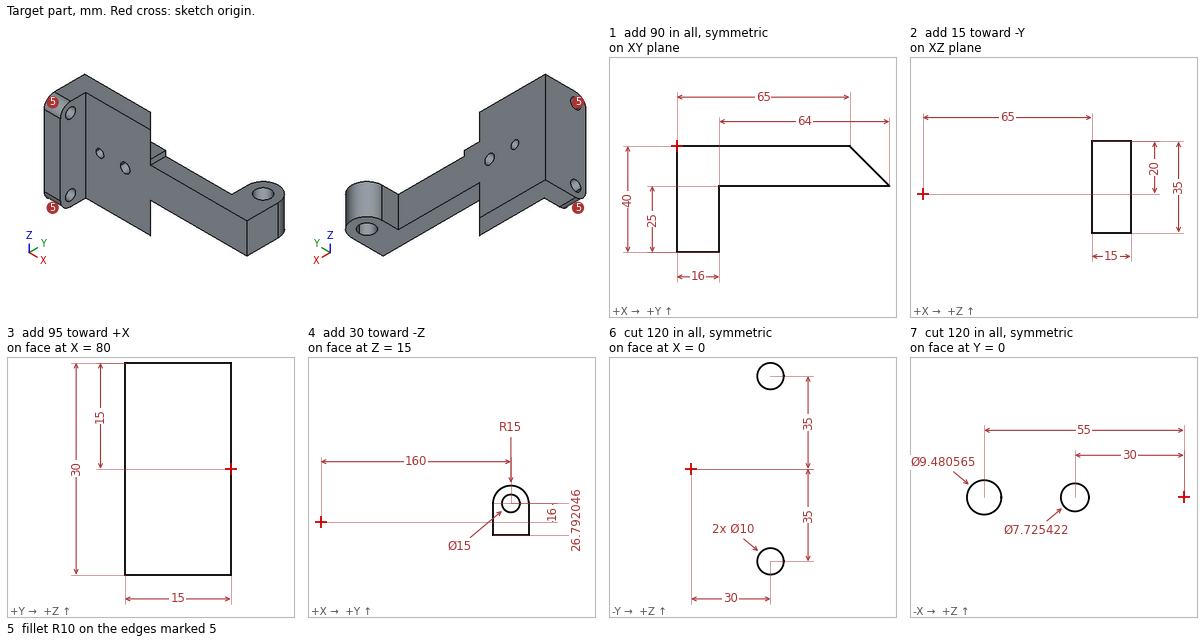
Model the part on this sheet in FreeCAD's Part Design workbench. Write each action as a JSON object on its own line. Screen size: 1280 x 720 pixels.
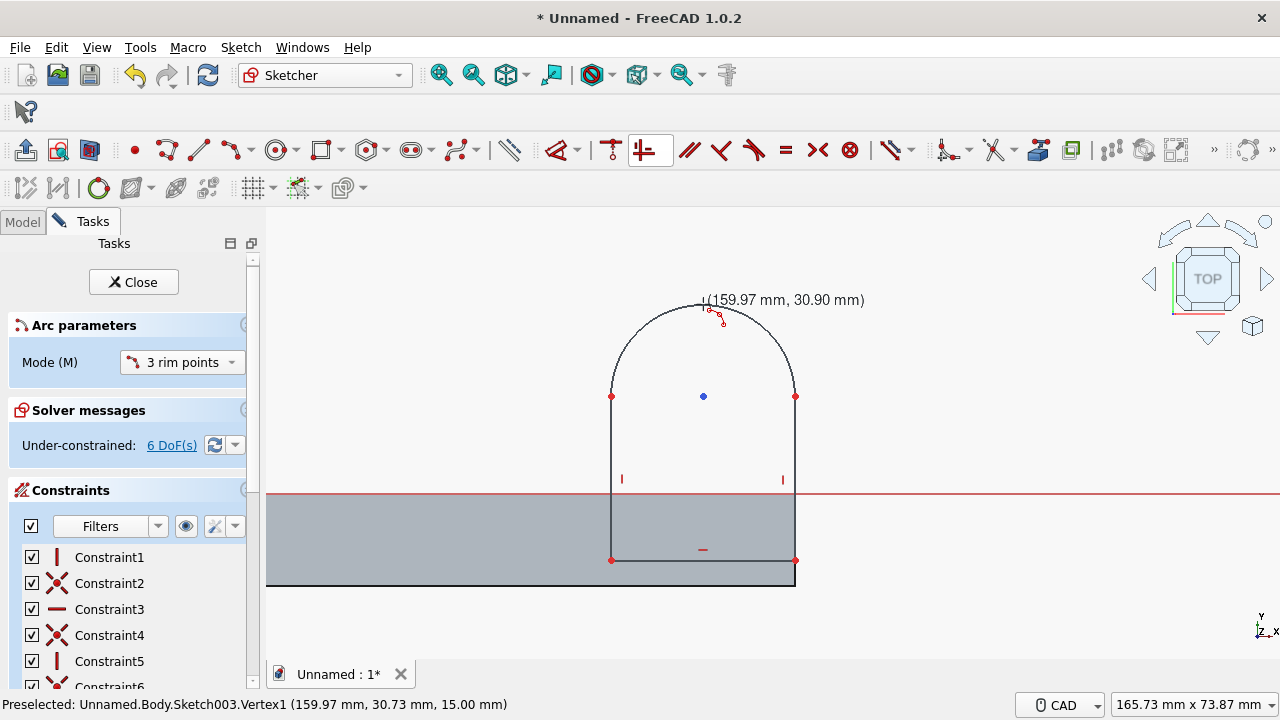
{"action": "key", "text": "g c"}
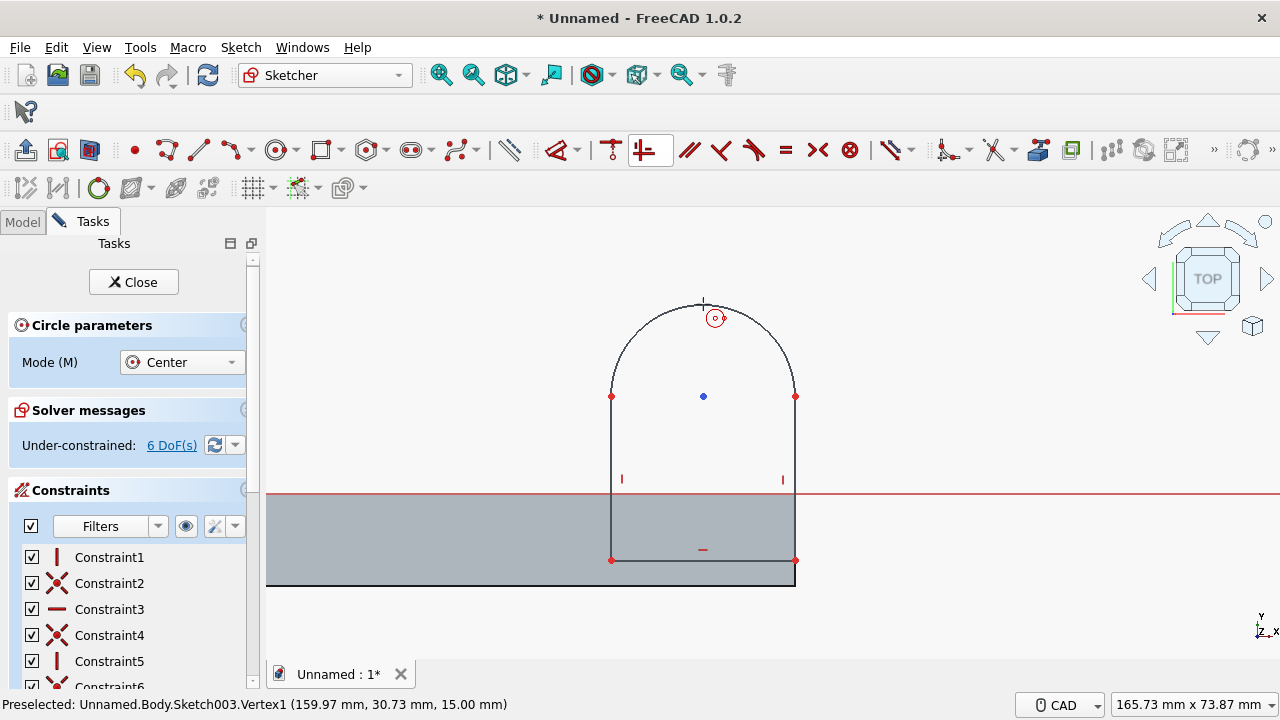
{"action": "left_click", "coordinate": [703, 396]}
{"action": "mouse_move", "coordinate": [736, 364]}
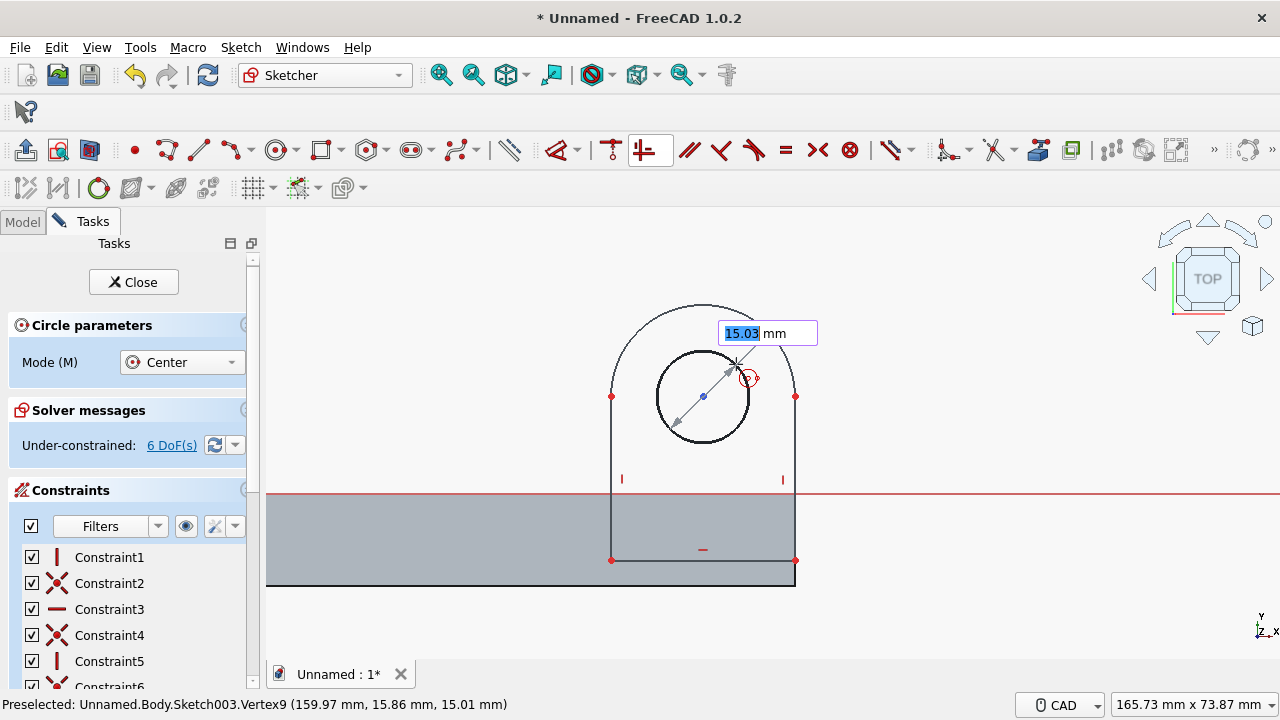
{"action": "type", "text": "15"}
{"action": "key", "text": "Return"}
{"action": "key", "text": "Escape"}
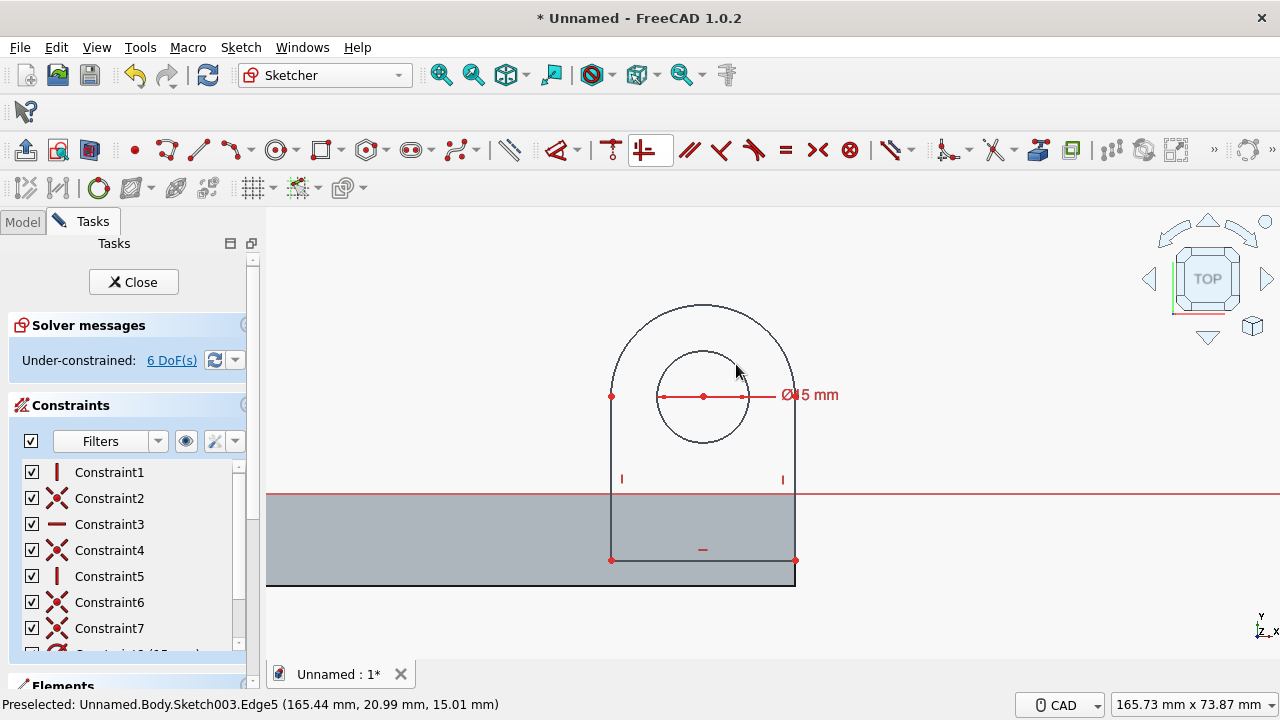
{"action": "left_click", "coordinate": [611, 446]}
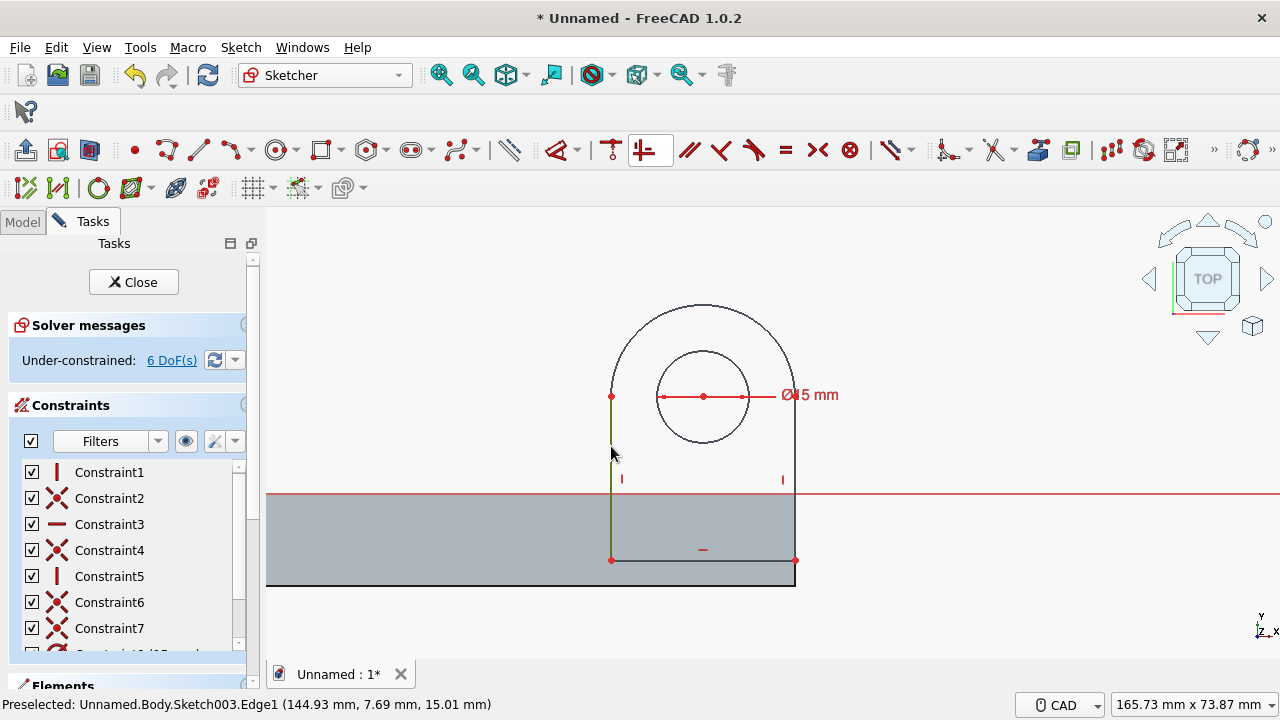
{"action": "left_click", "coordinate": [757, 323]}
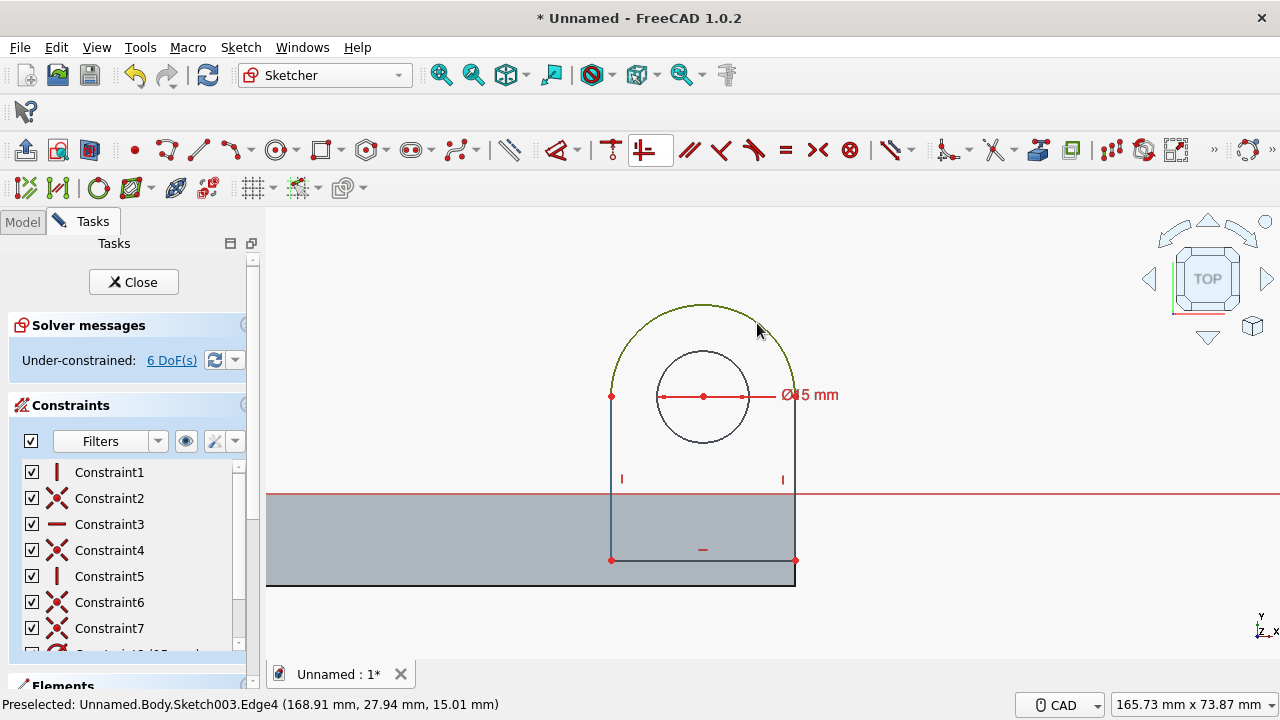
{"action": "left_click", "coordinate": [754, 150]}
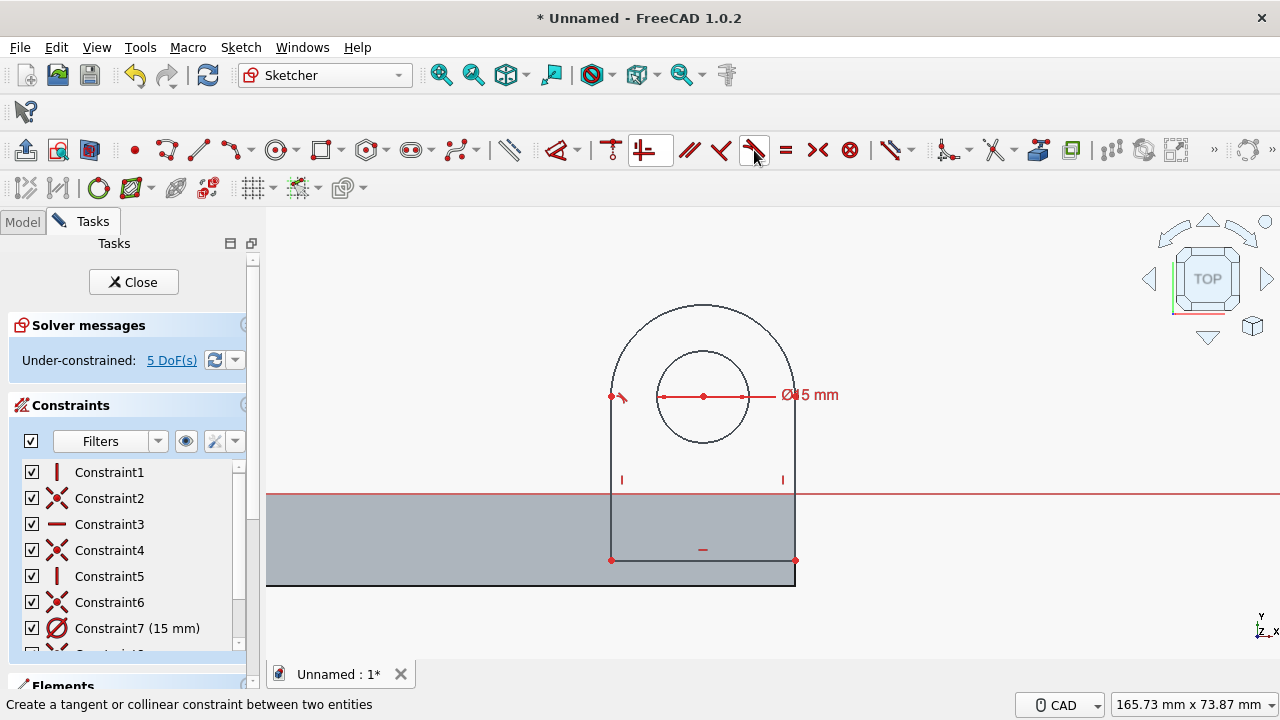
{"action": "left_click", "coordinate": [795, 512]}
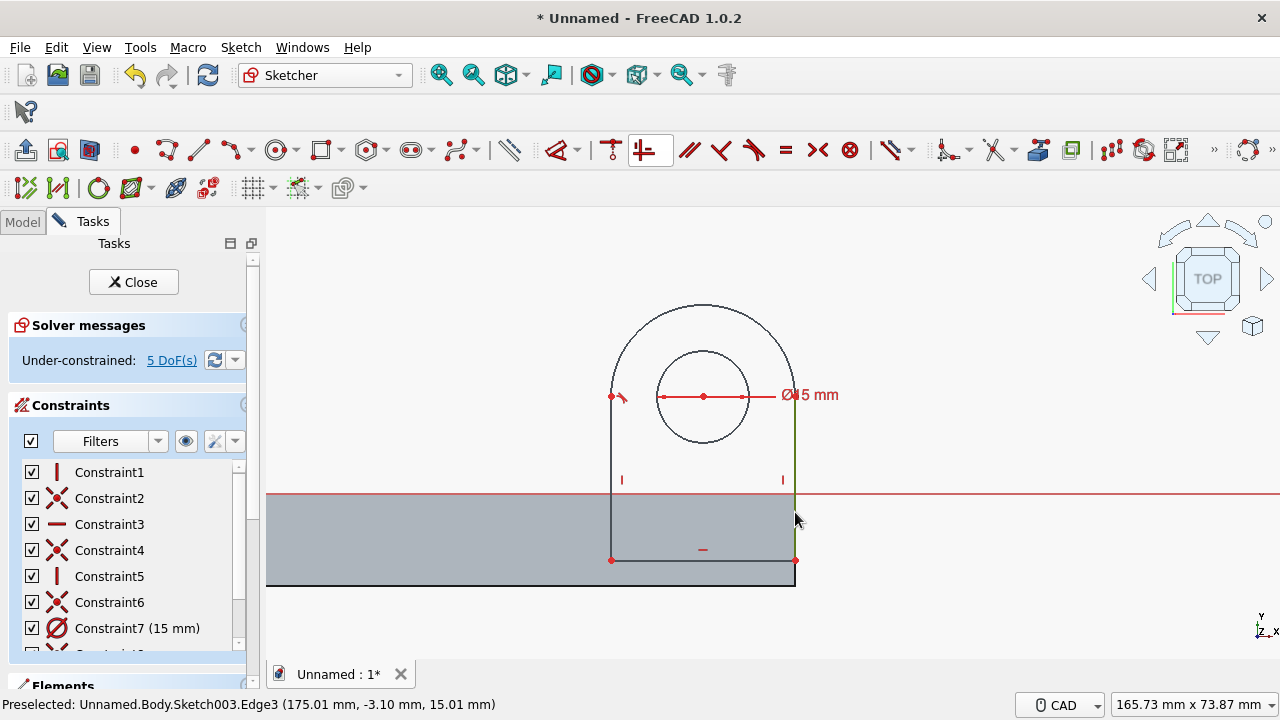
{"action": "left_click", "coordinate": [757, 323]}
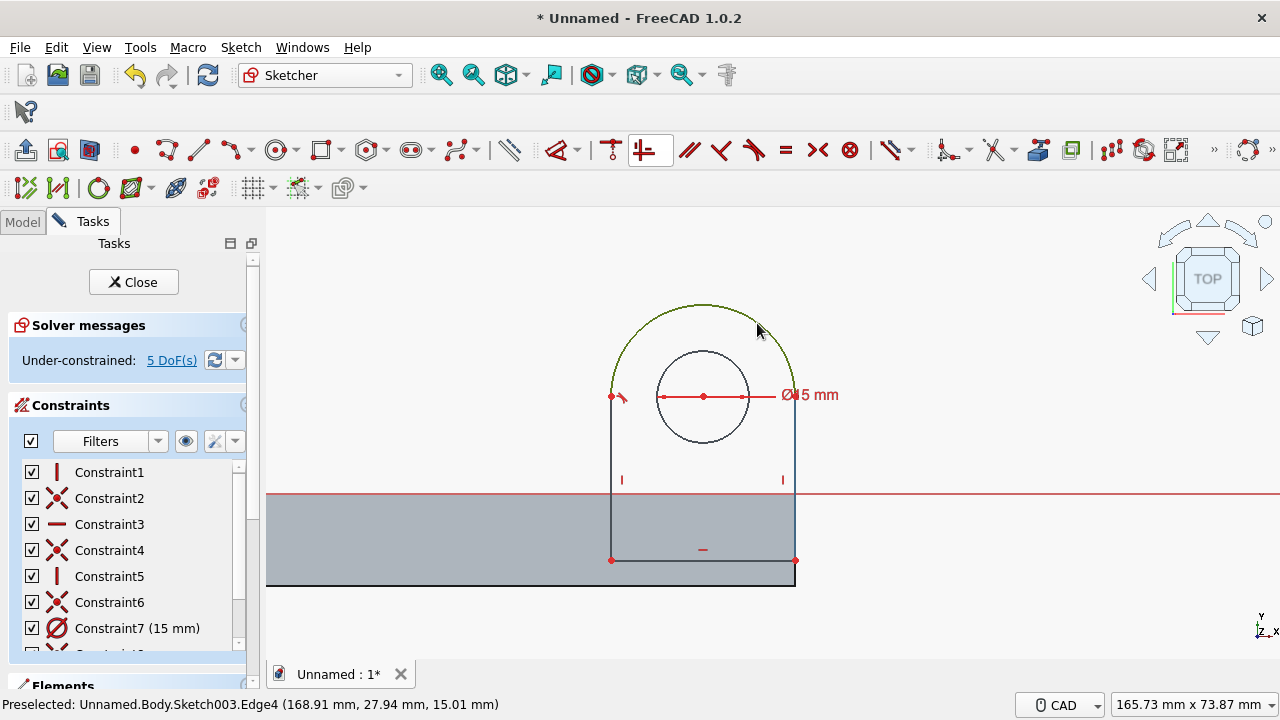
{"action": "key", "text": "t"}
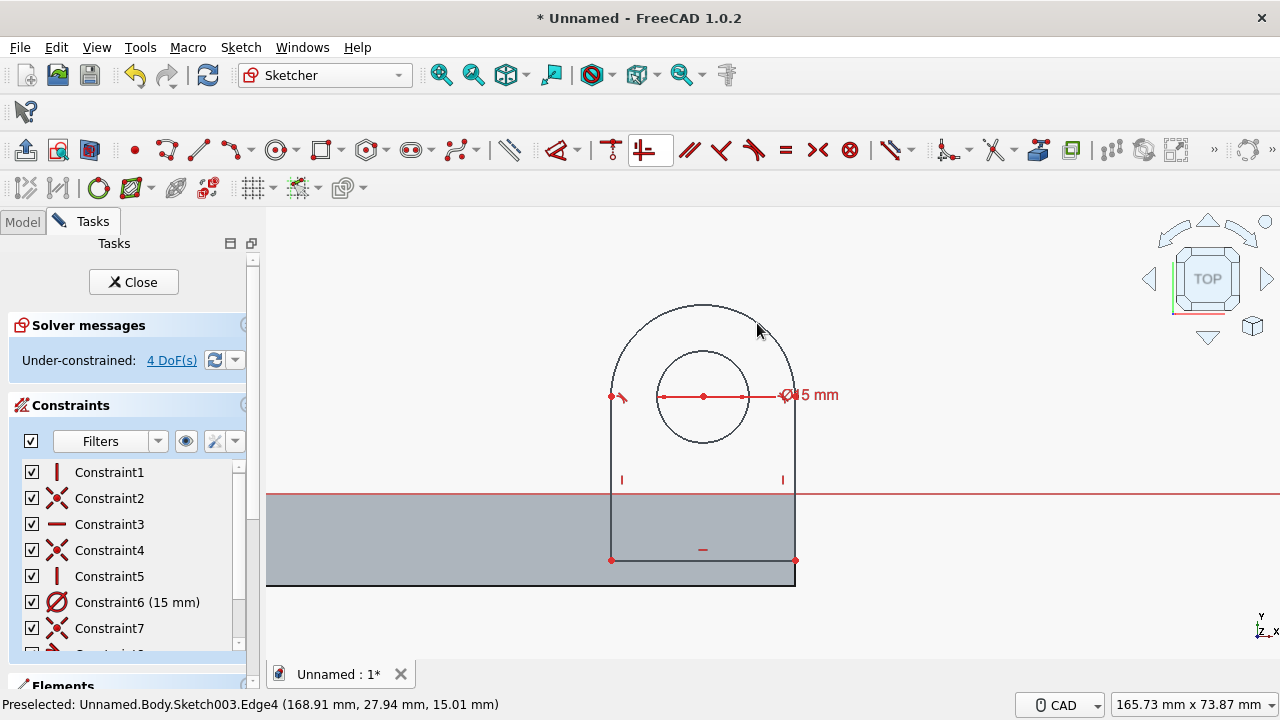
{"action": "left_click", "coordinate": [556, 150]}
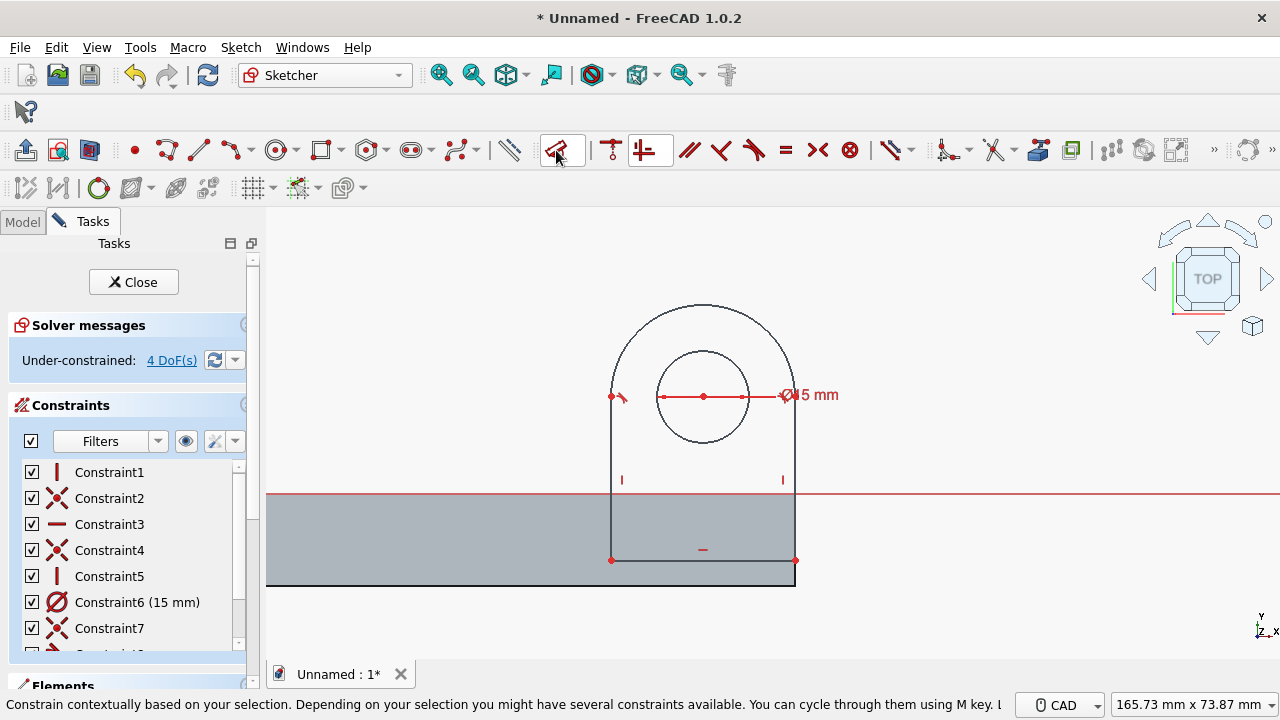
{"action": "left_click", "coordinate": [757, 323]}
{"action": "left_click", "coordinate": [776, 297]}